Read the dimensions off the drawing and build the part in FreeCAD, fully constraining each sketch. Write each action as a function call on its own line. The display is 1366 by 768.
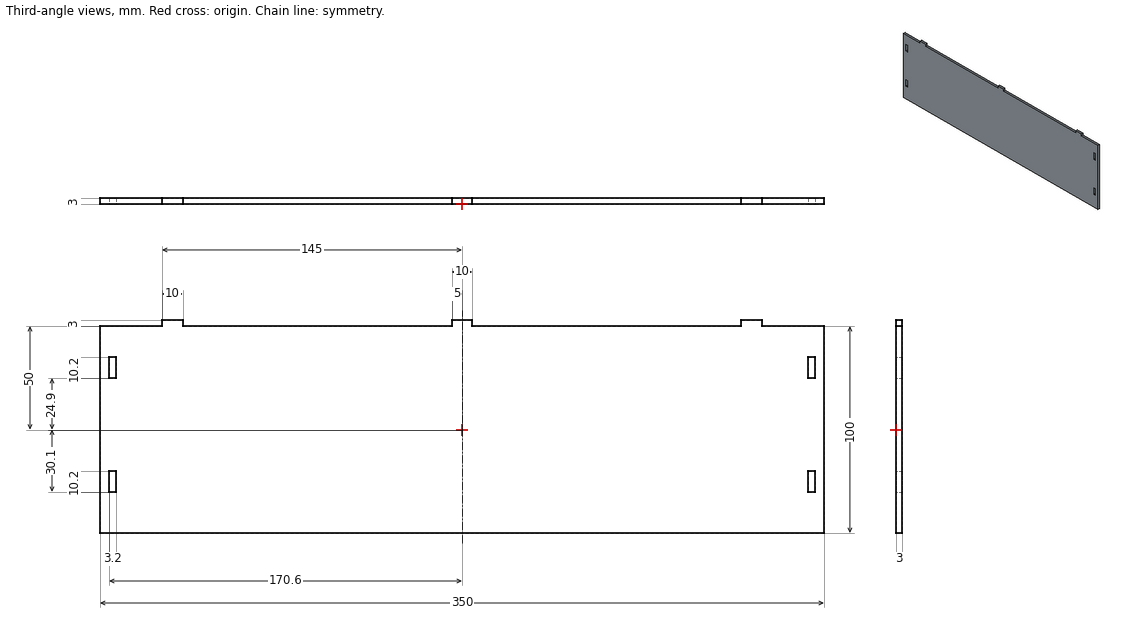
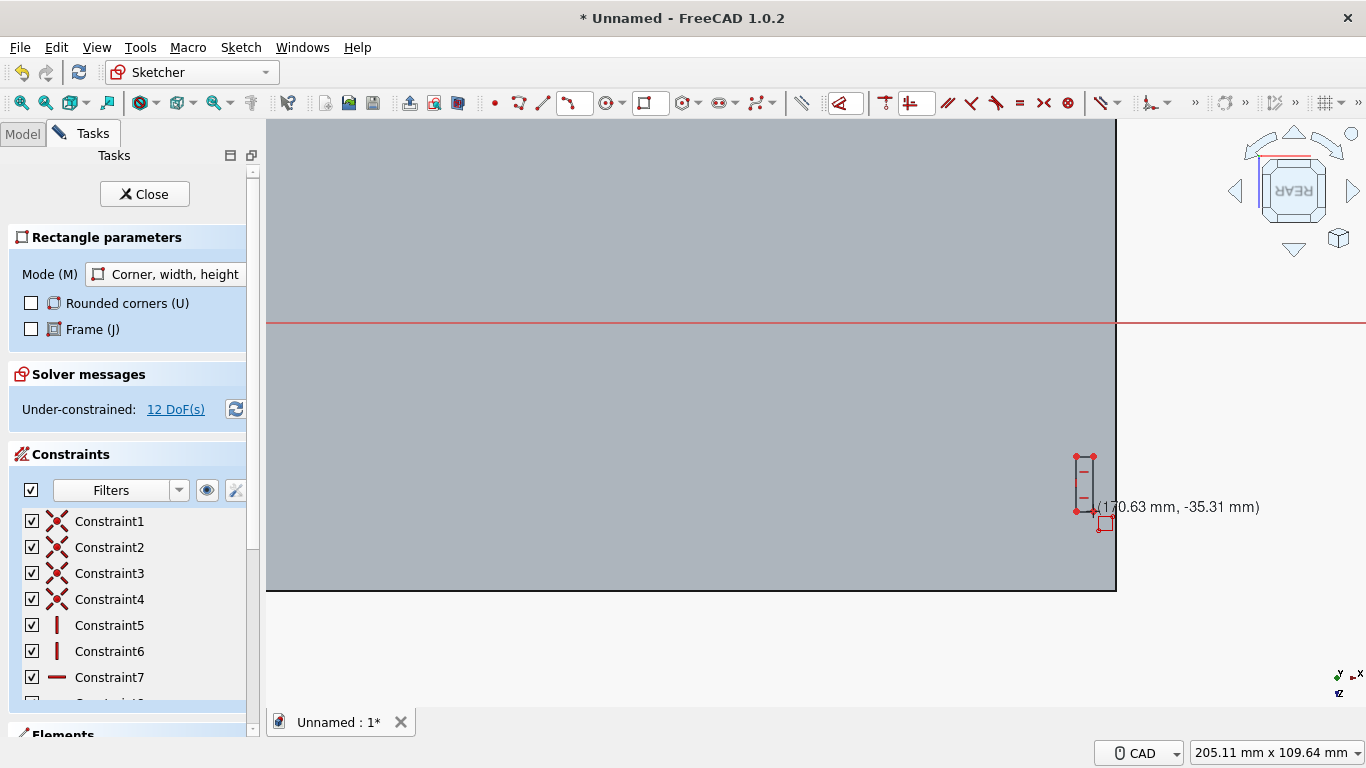
click(1076, 161)
click(1093, 216)
key(Escape)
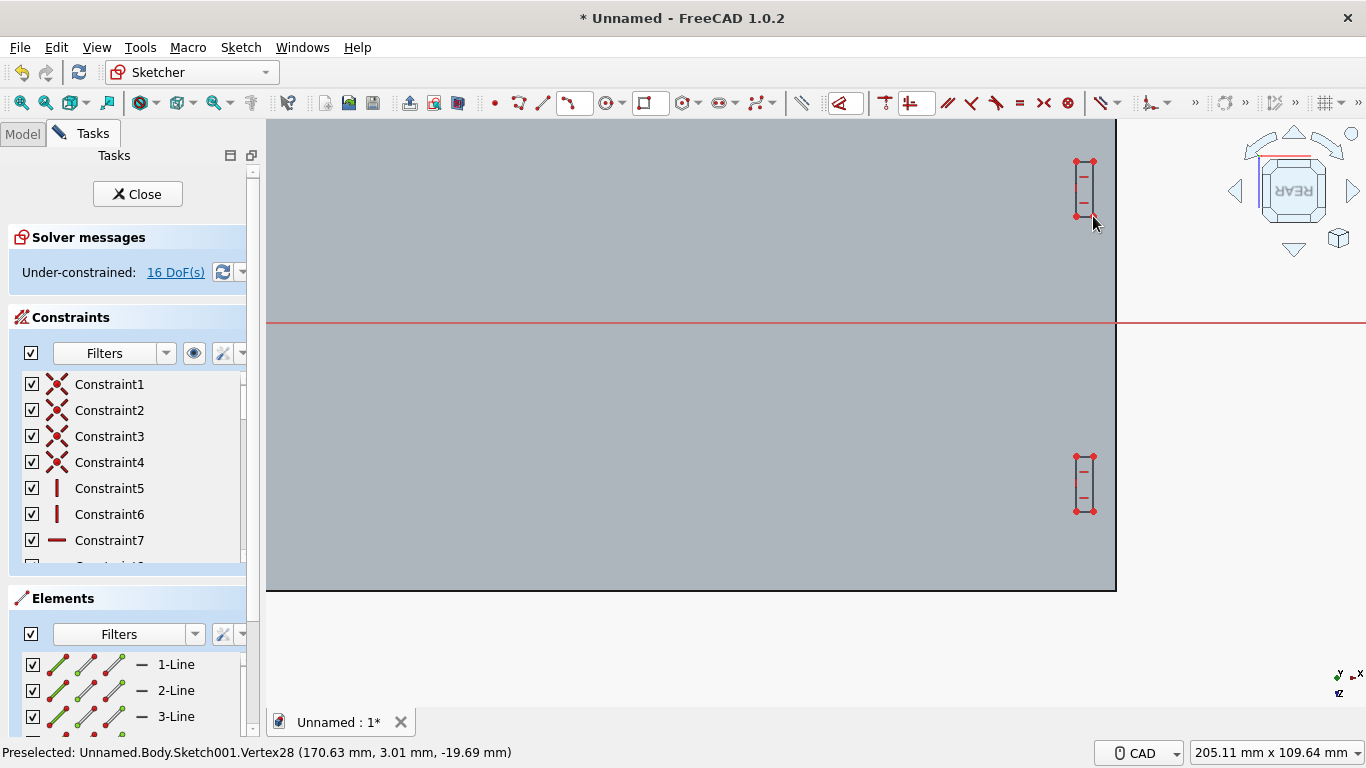
scroll(1079, 458, down, 5)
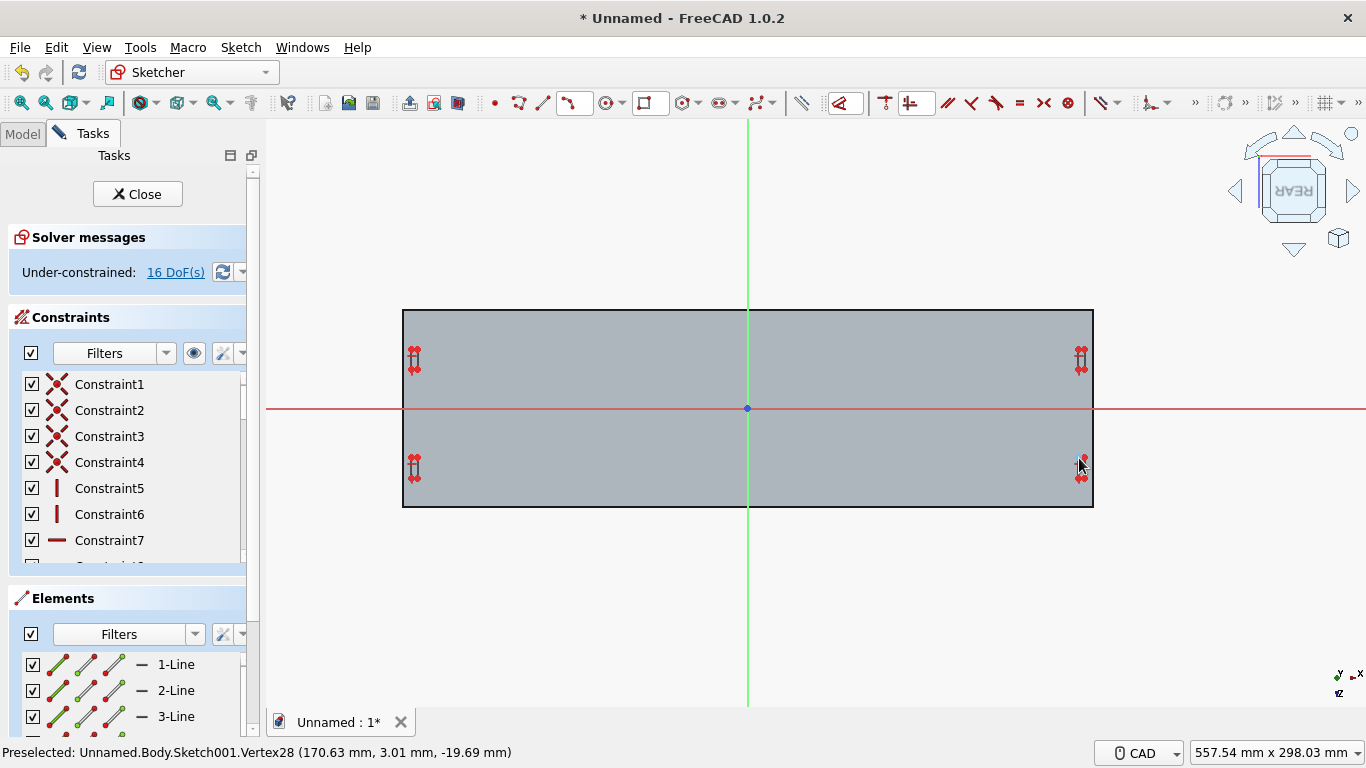
scroll(418, 458, up, 4)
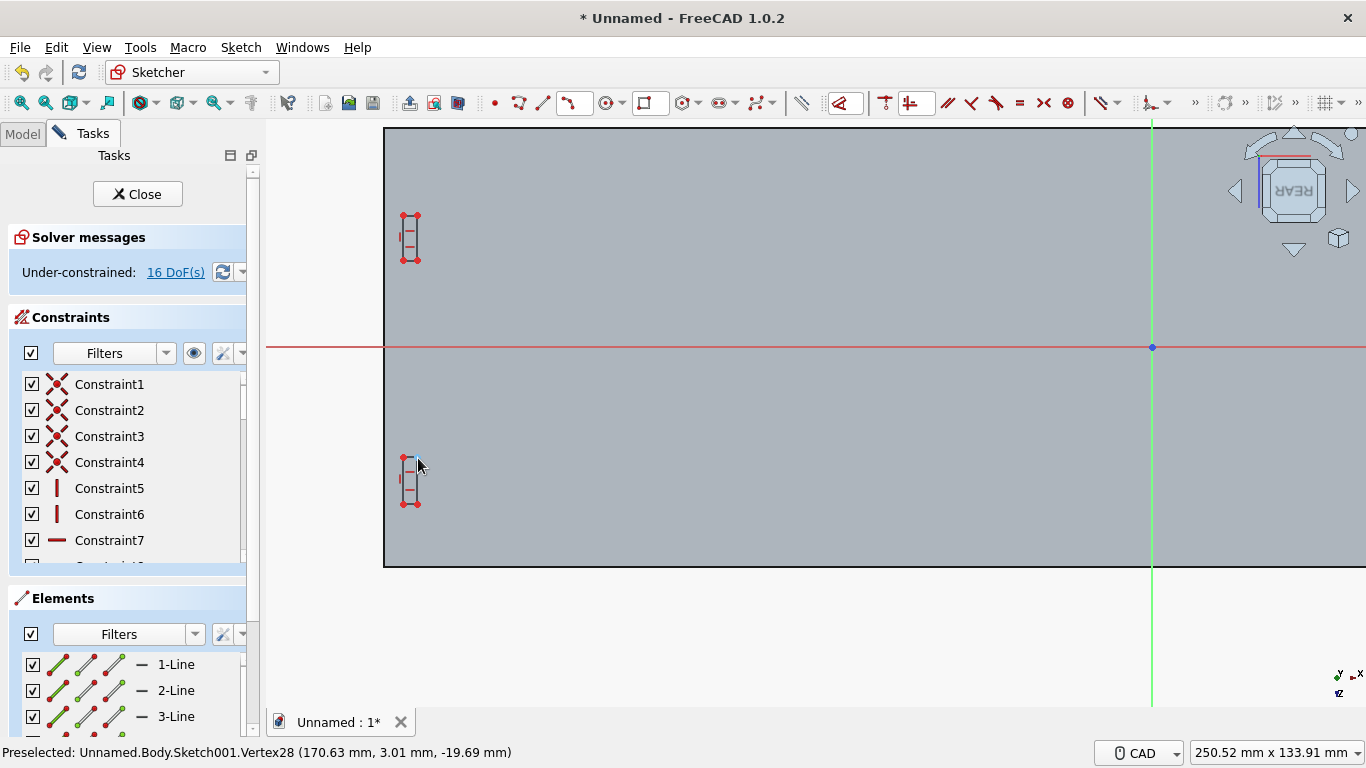
click(417, 457)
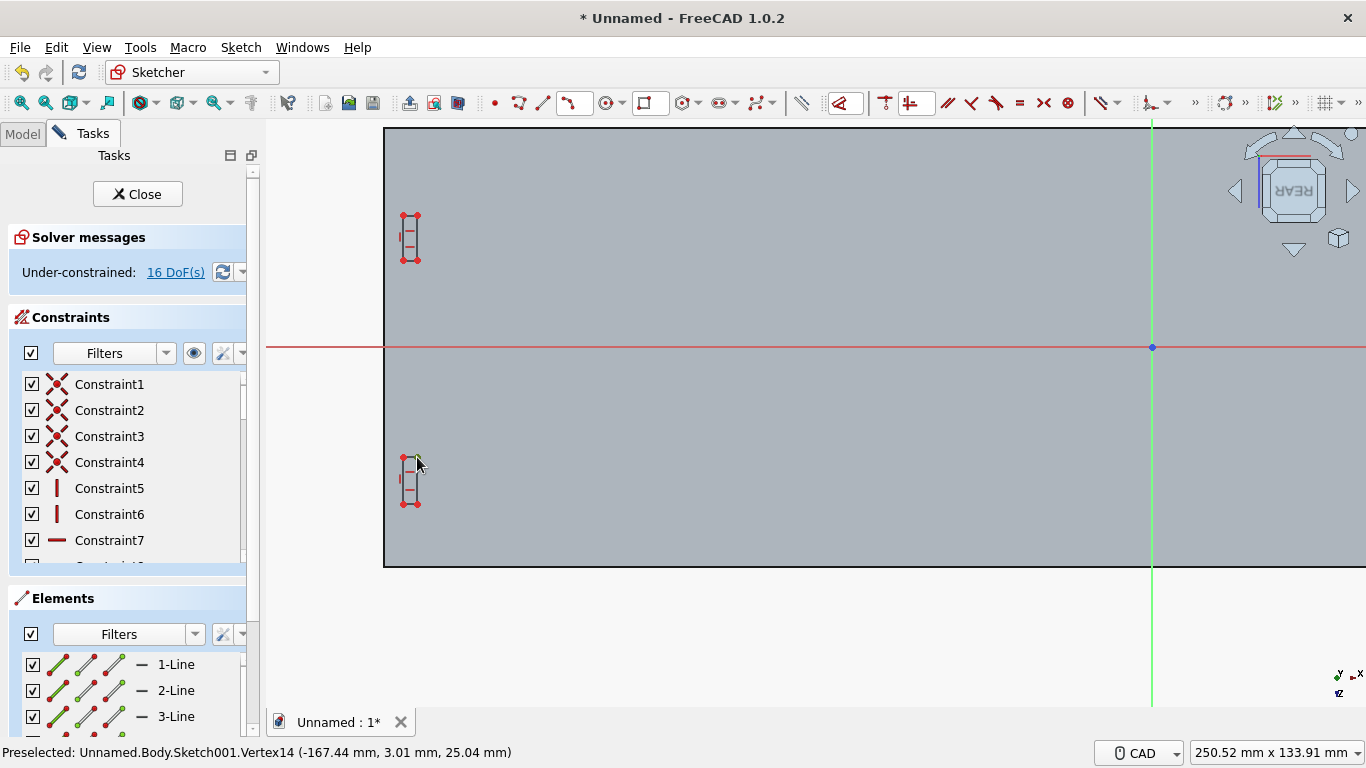
scroll(417, 458, down, 4)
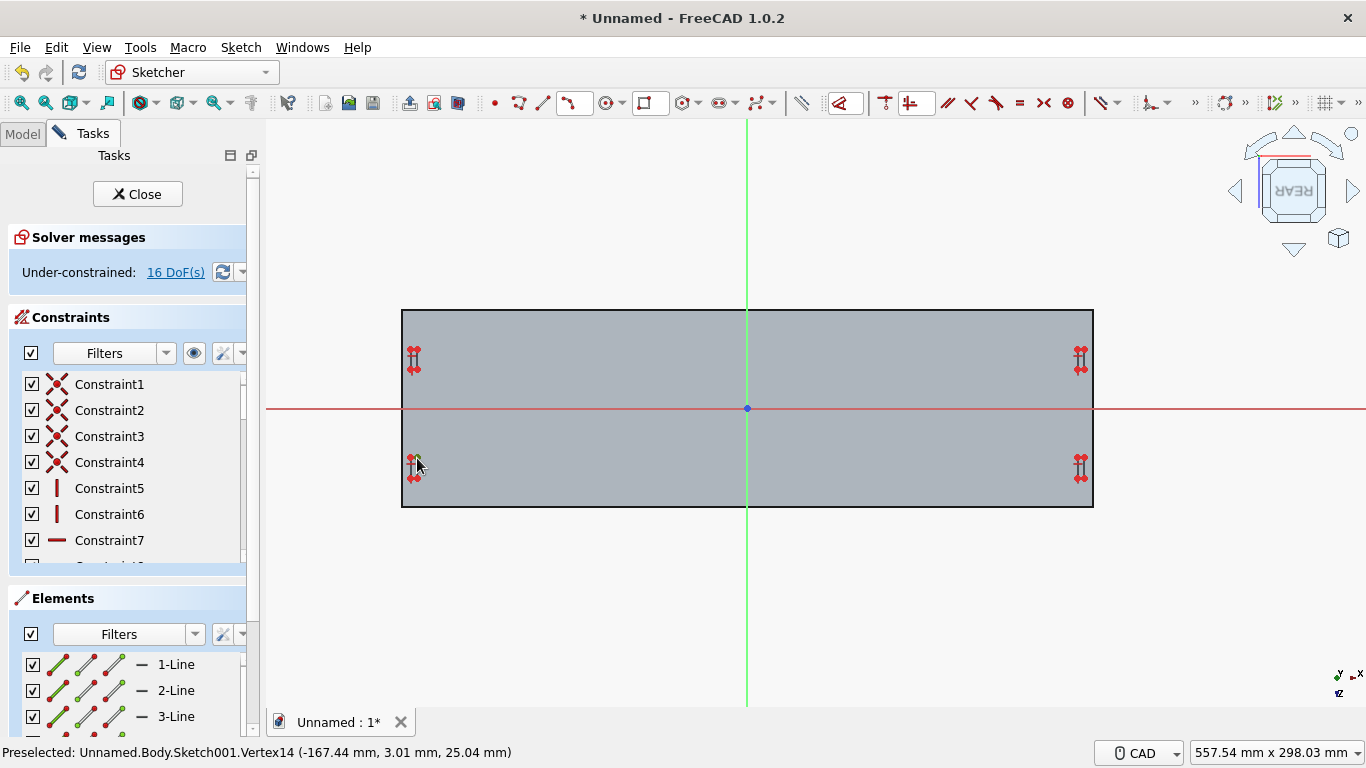
scroll(1078, 458, up, 4)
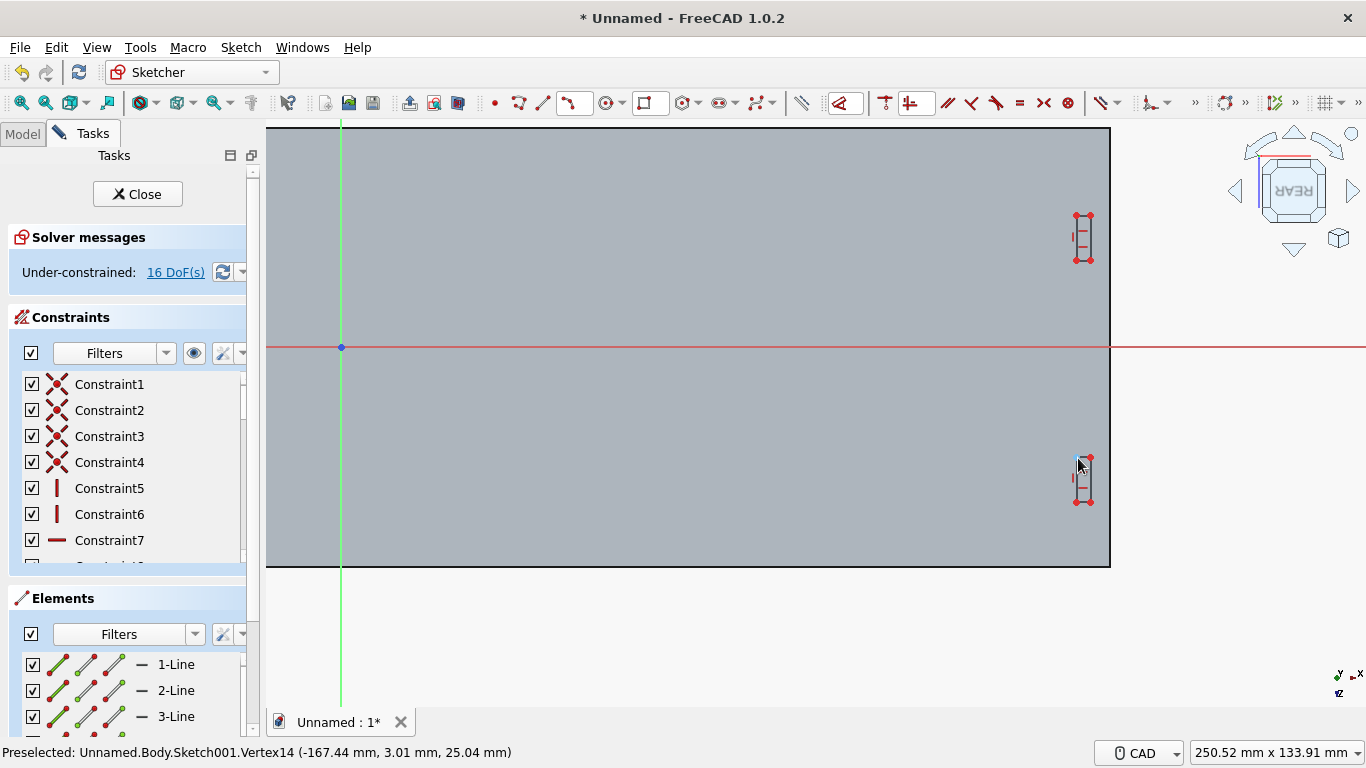
click(1077, 457)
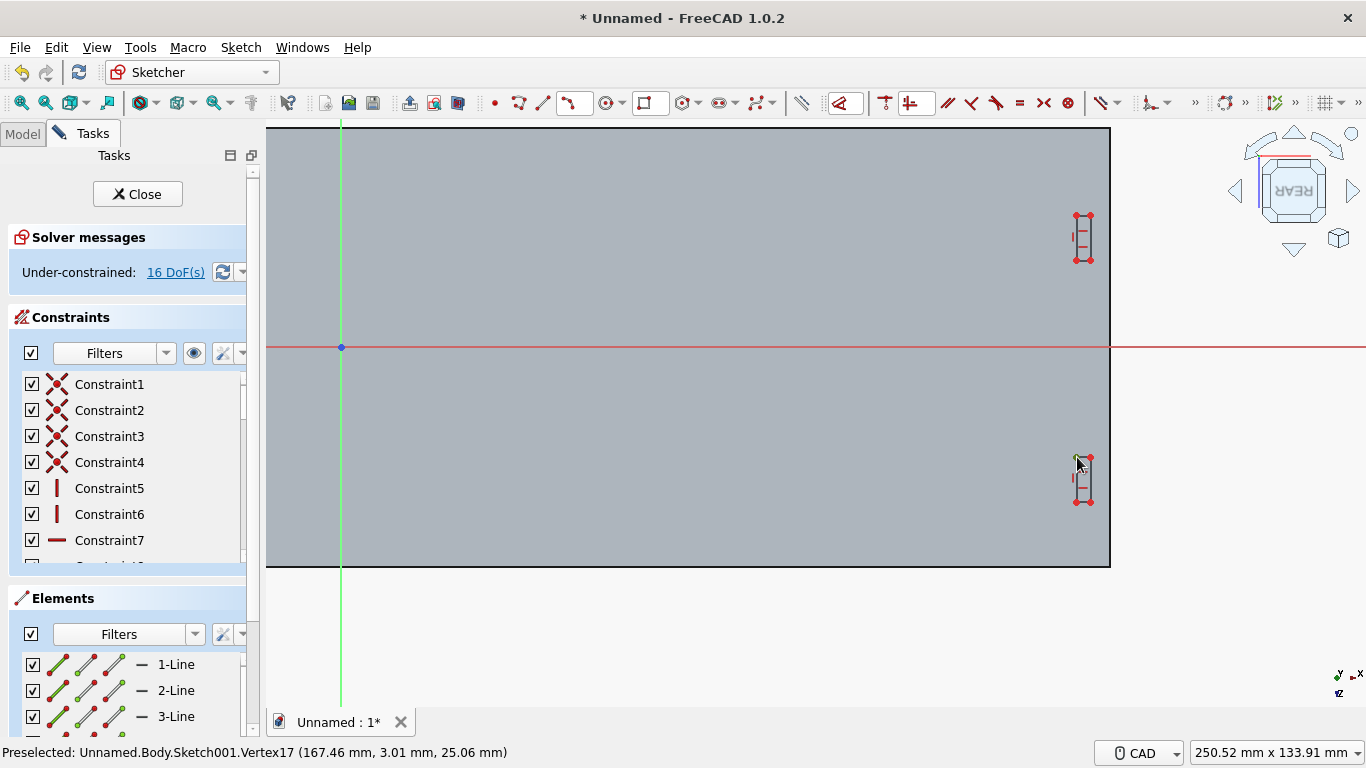
click(341, 641)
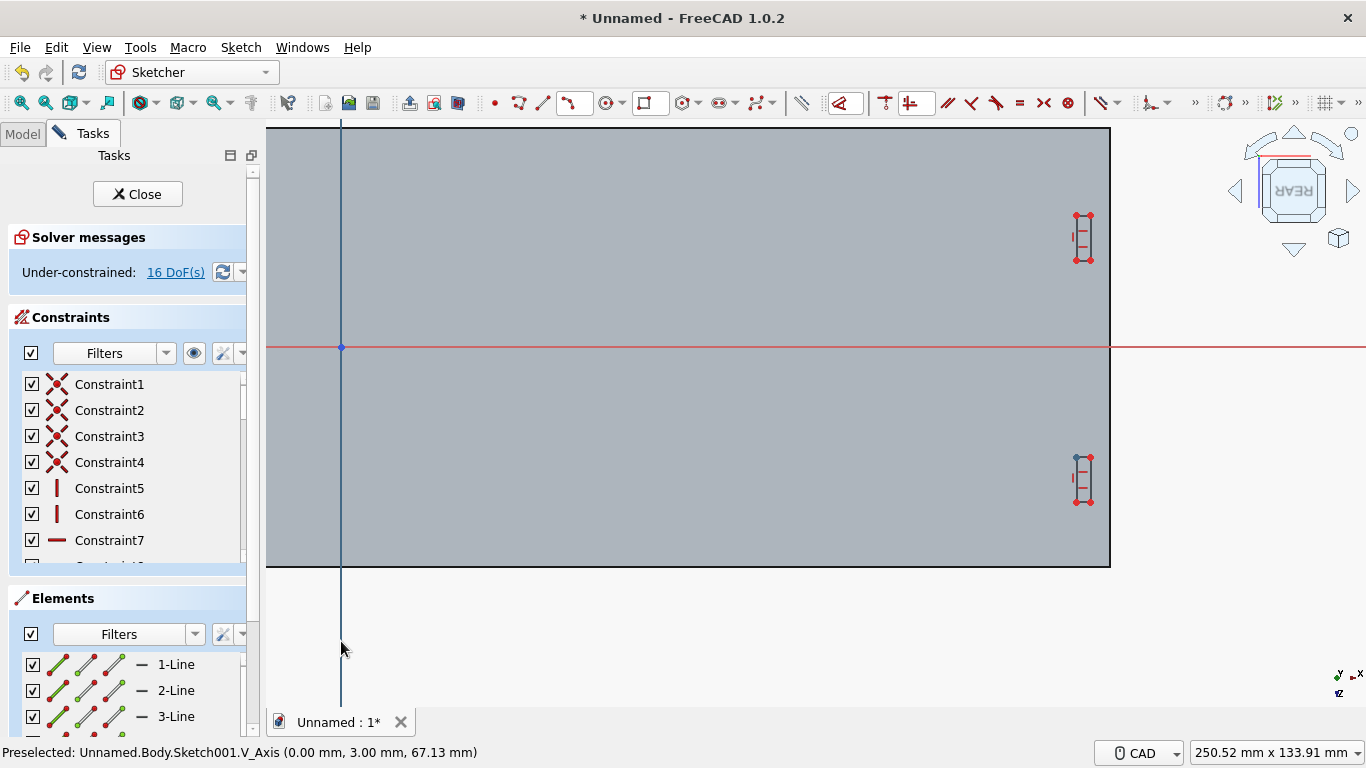
click(1044, 104)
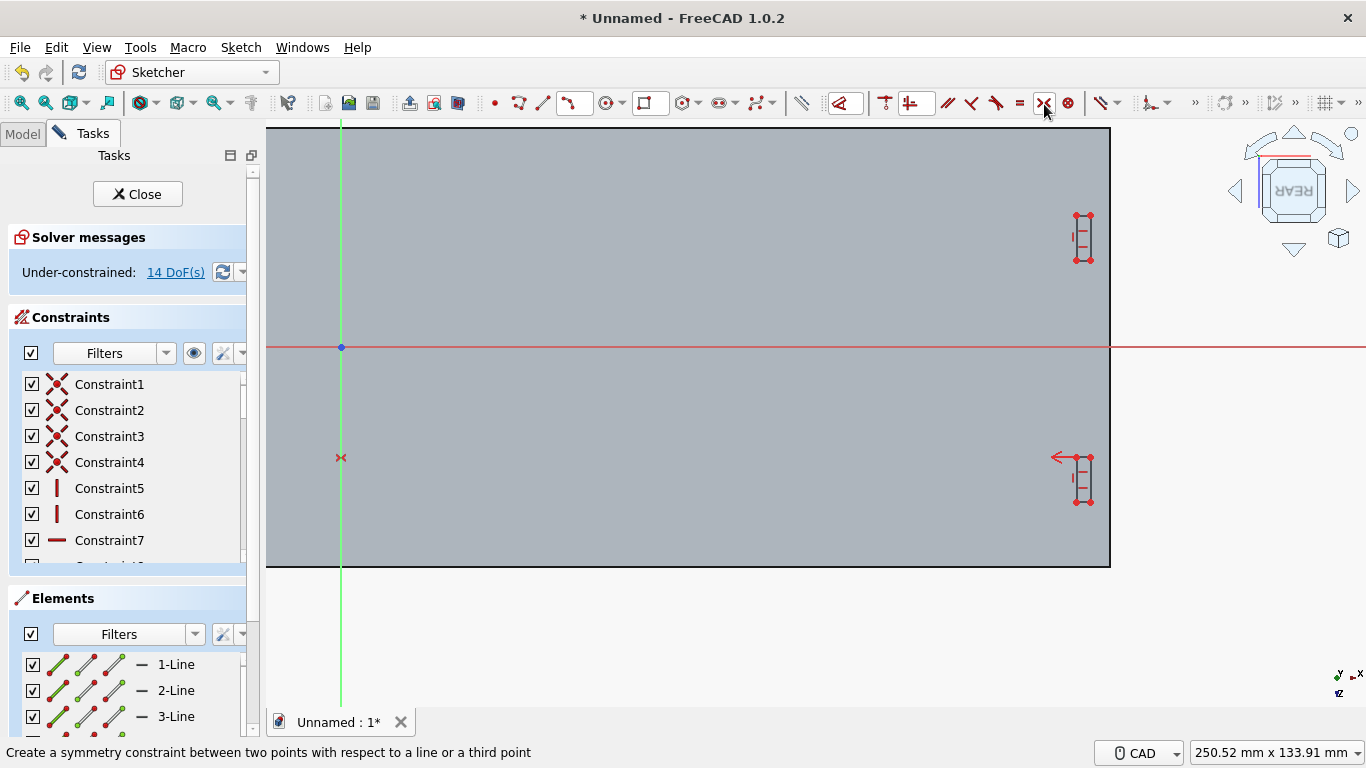
scroll(1079, 458, down, 4)